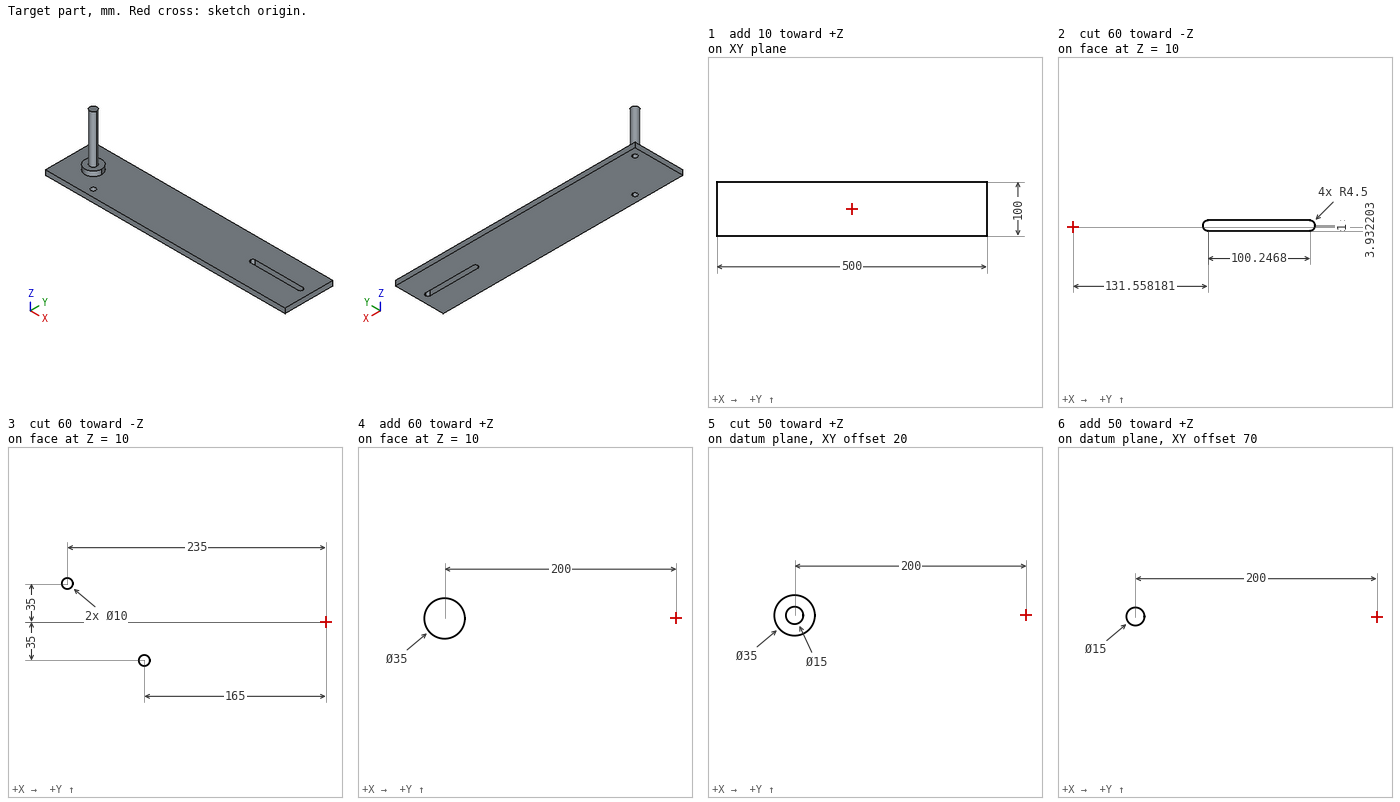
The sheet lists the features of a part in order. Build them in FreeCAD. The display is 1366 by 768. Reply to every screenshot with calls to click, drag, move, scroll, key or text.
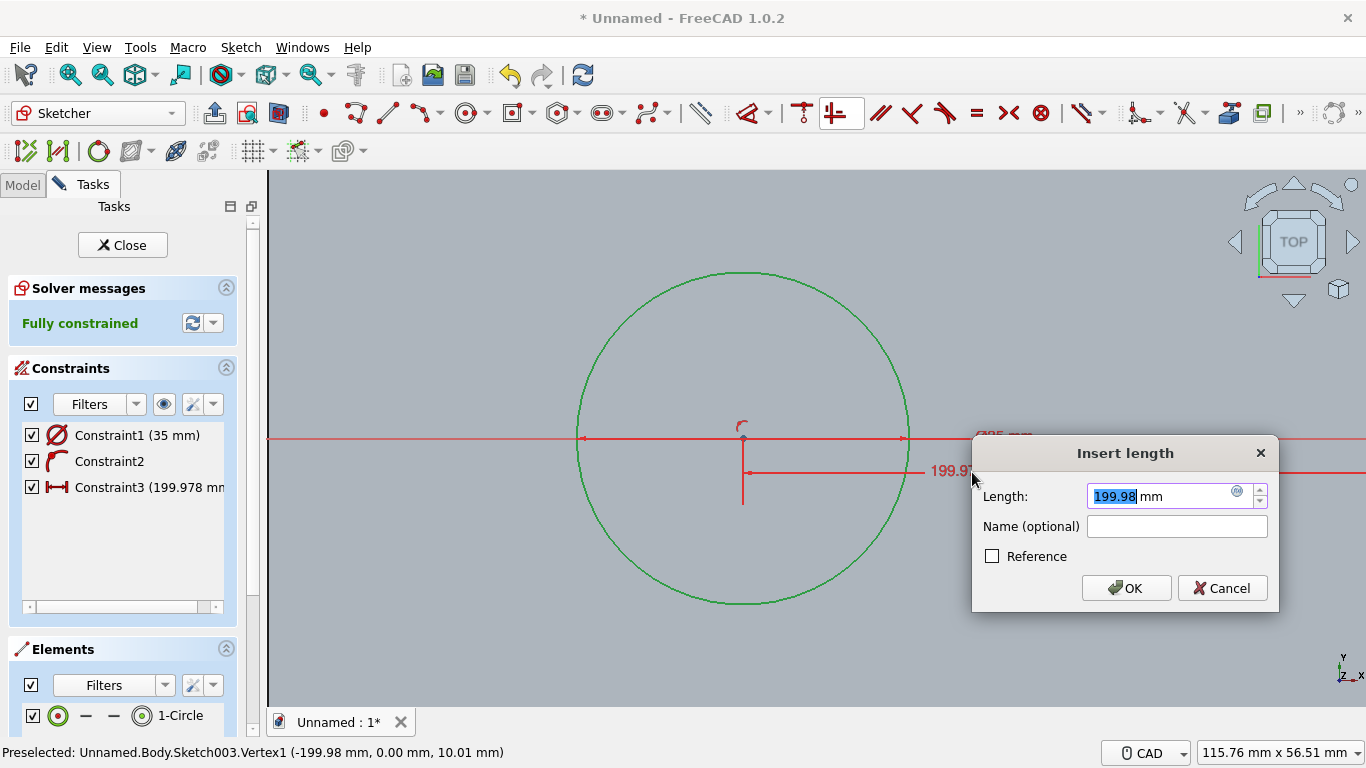
text(200)
key(Return)
key(Escape)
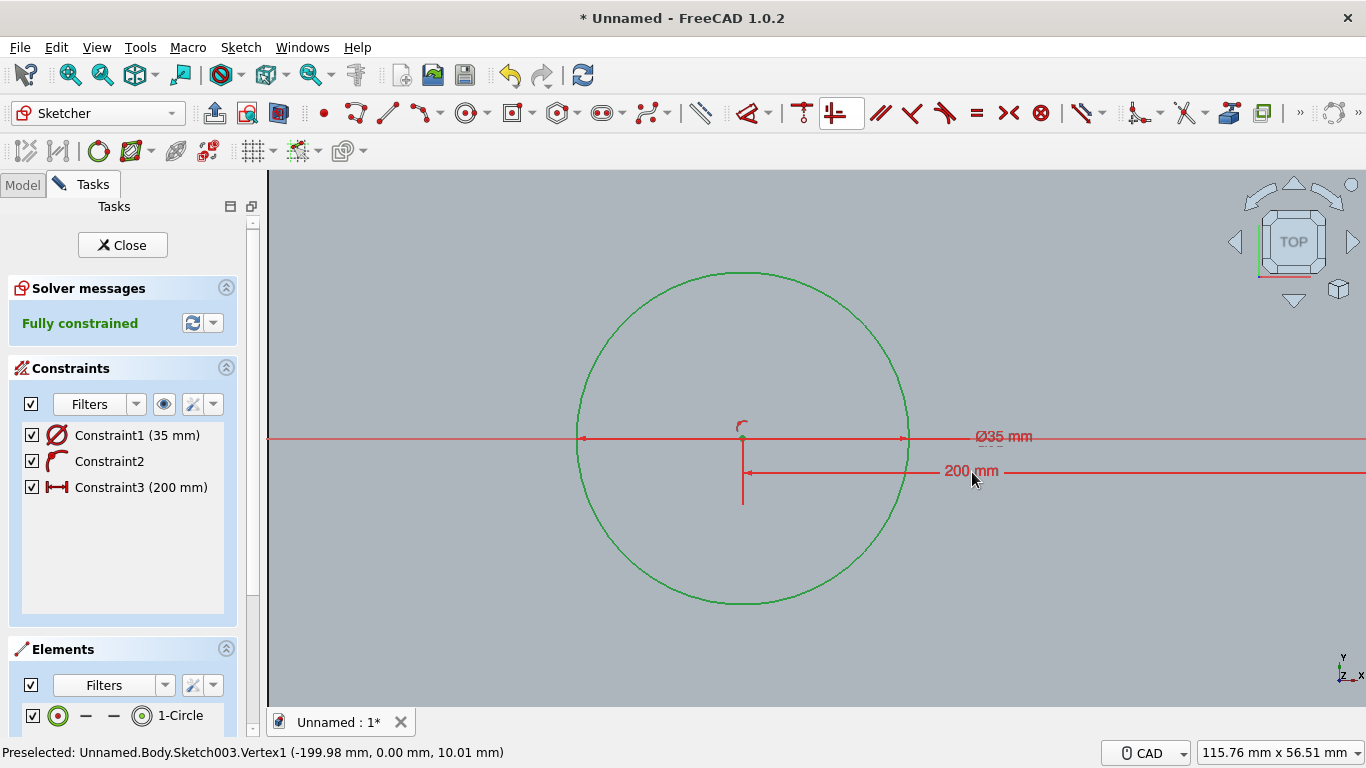
click(123, 245)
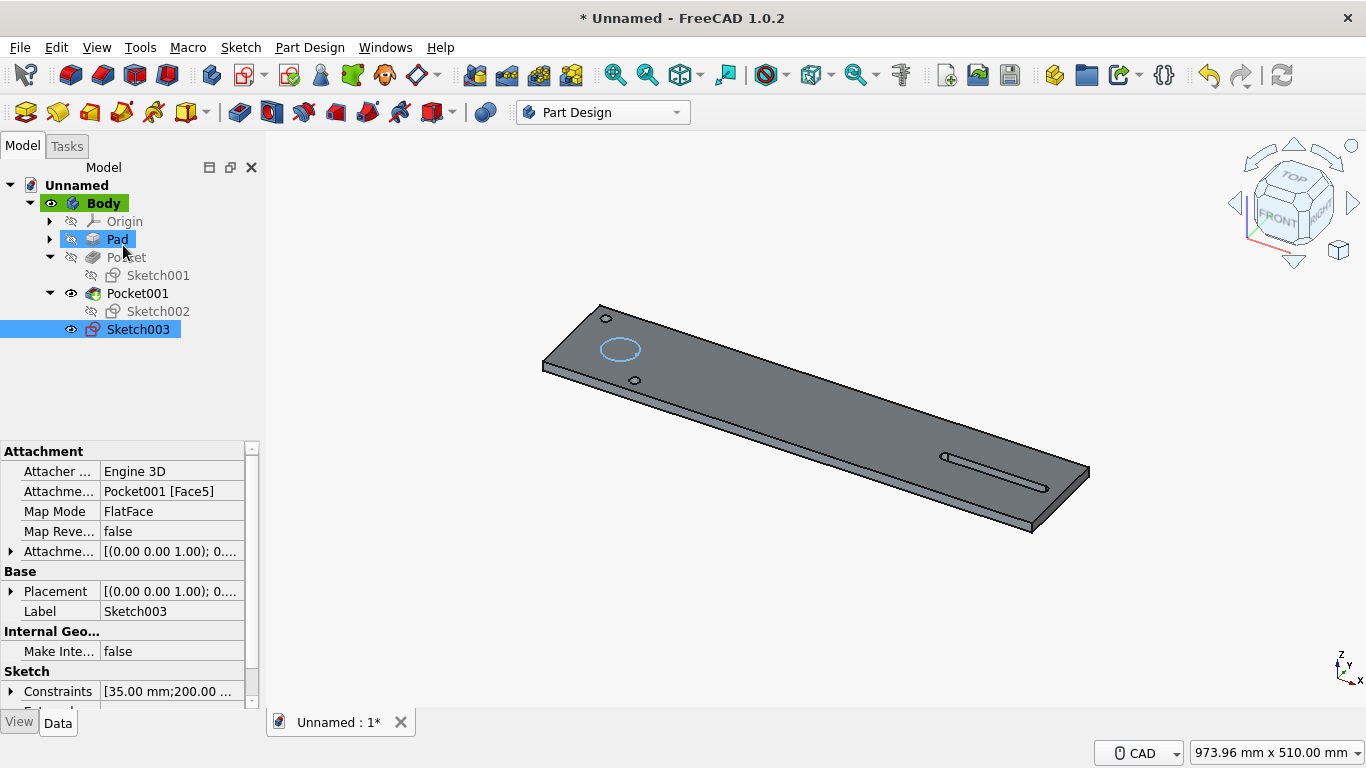
click(26, 112)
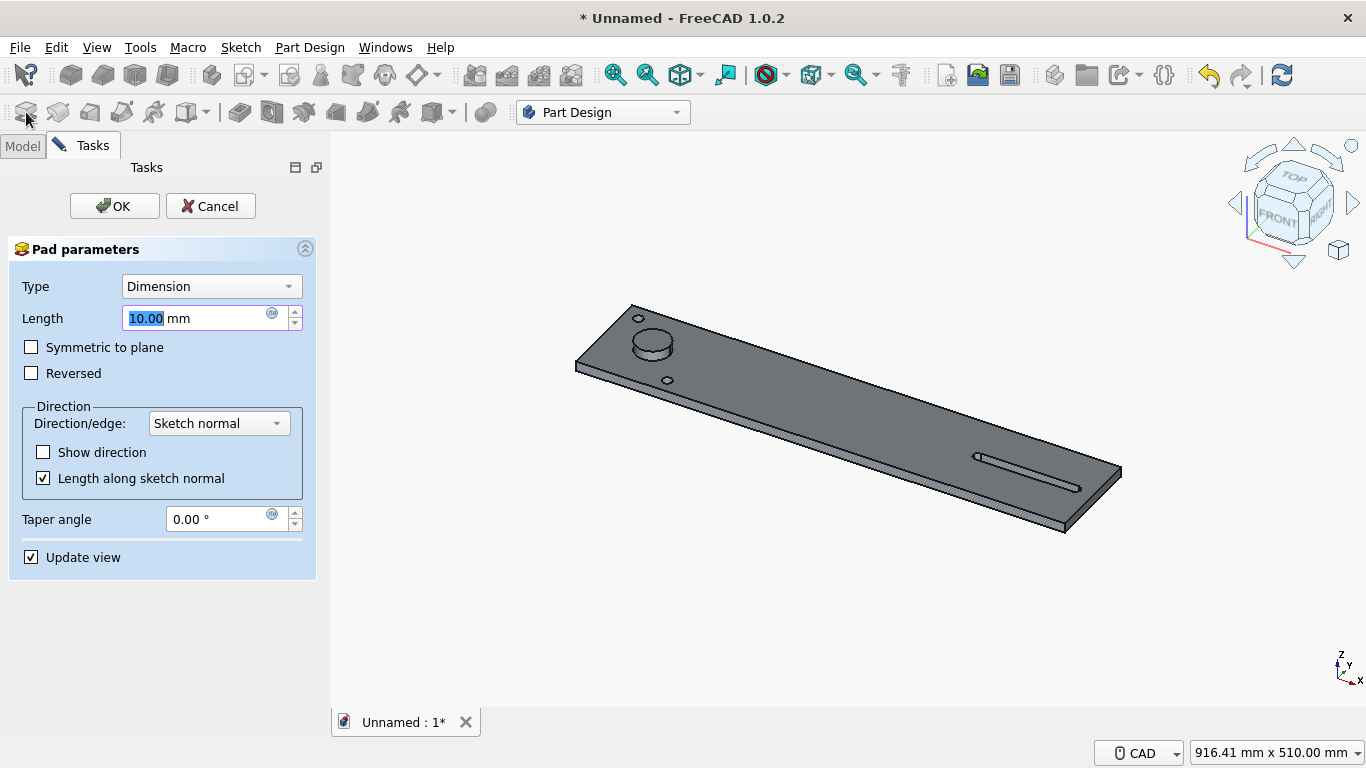
text(60)
key(Tab)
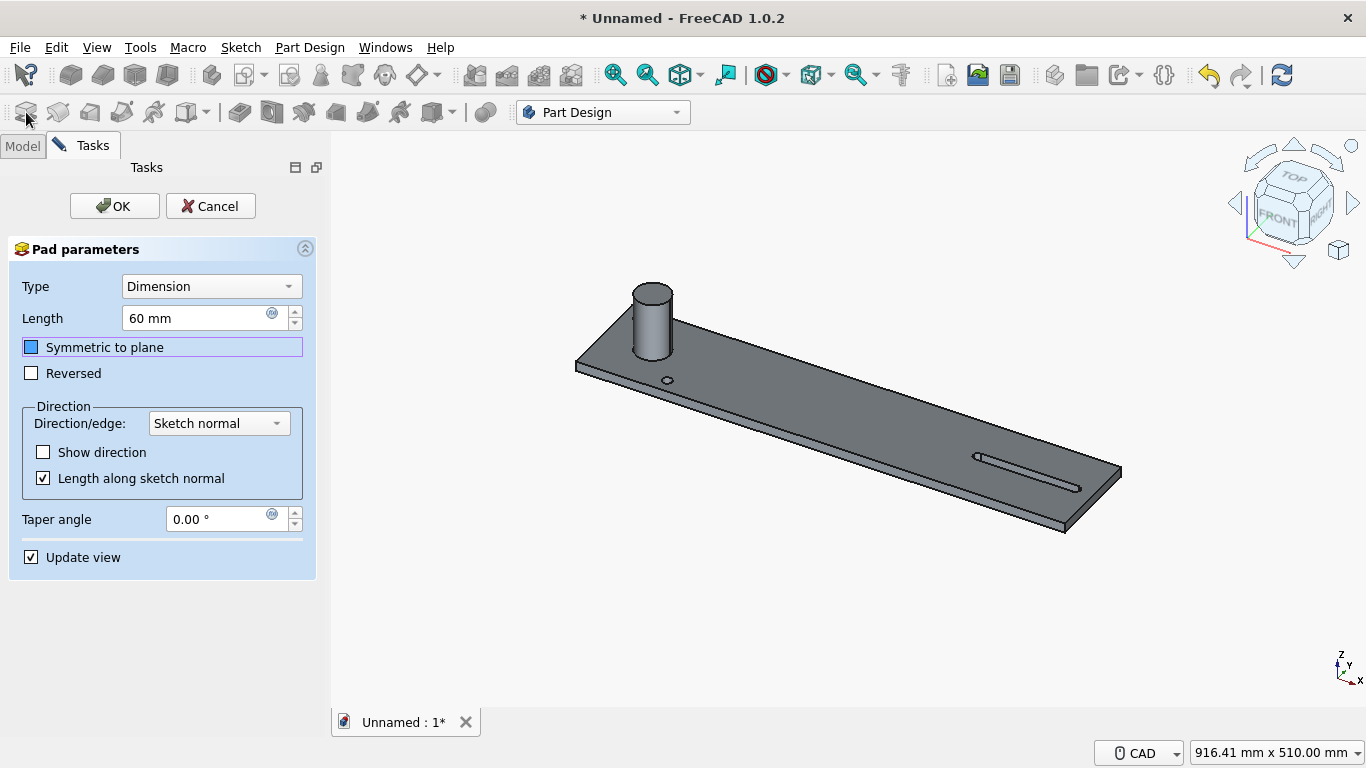
click(115, 206)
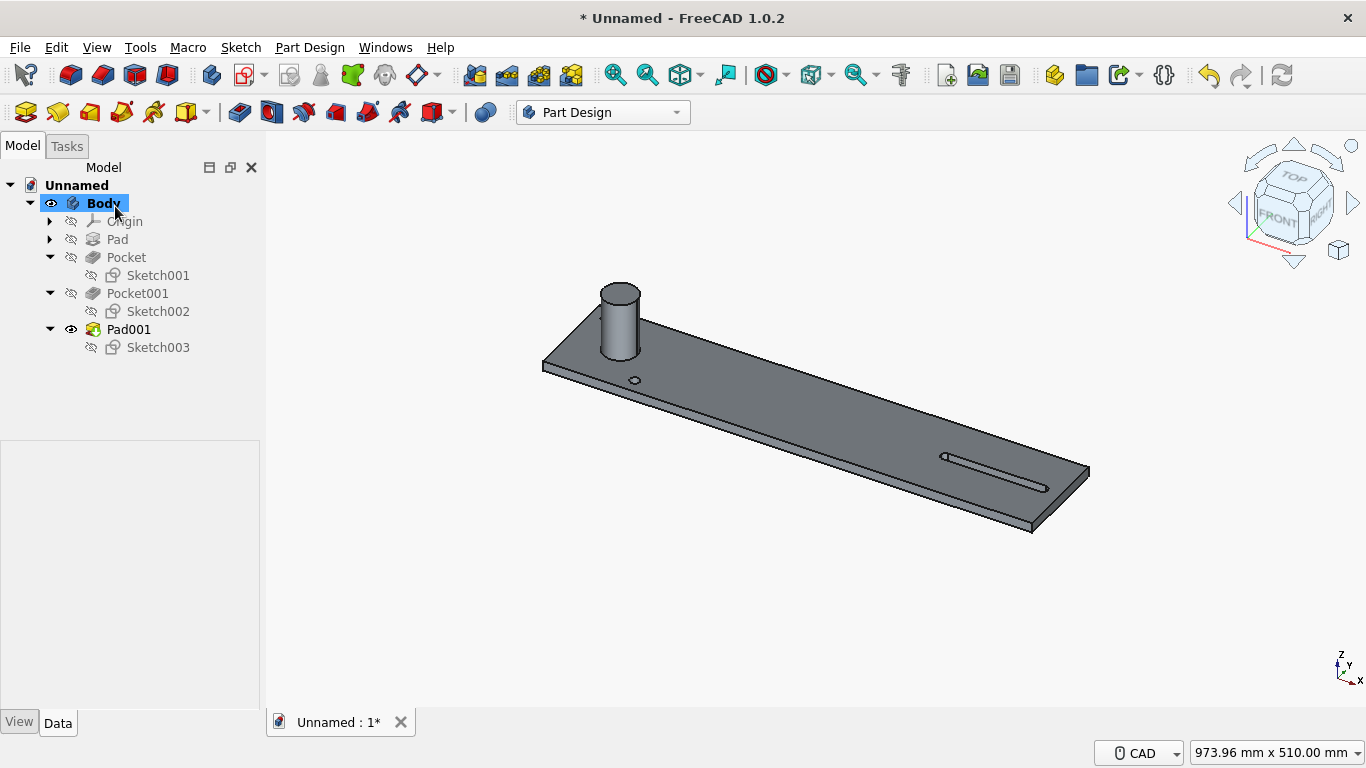
click(50, 221)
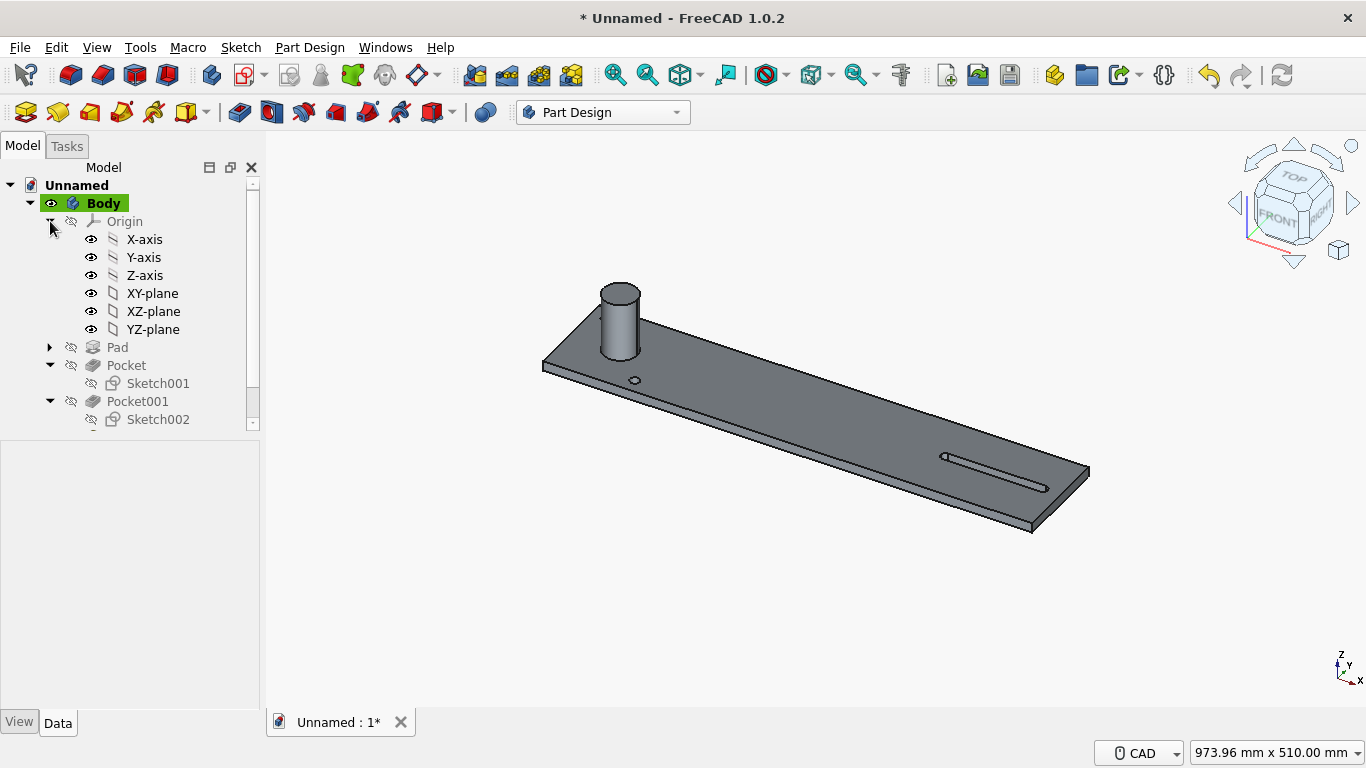
click(136, 293)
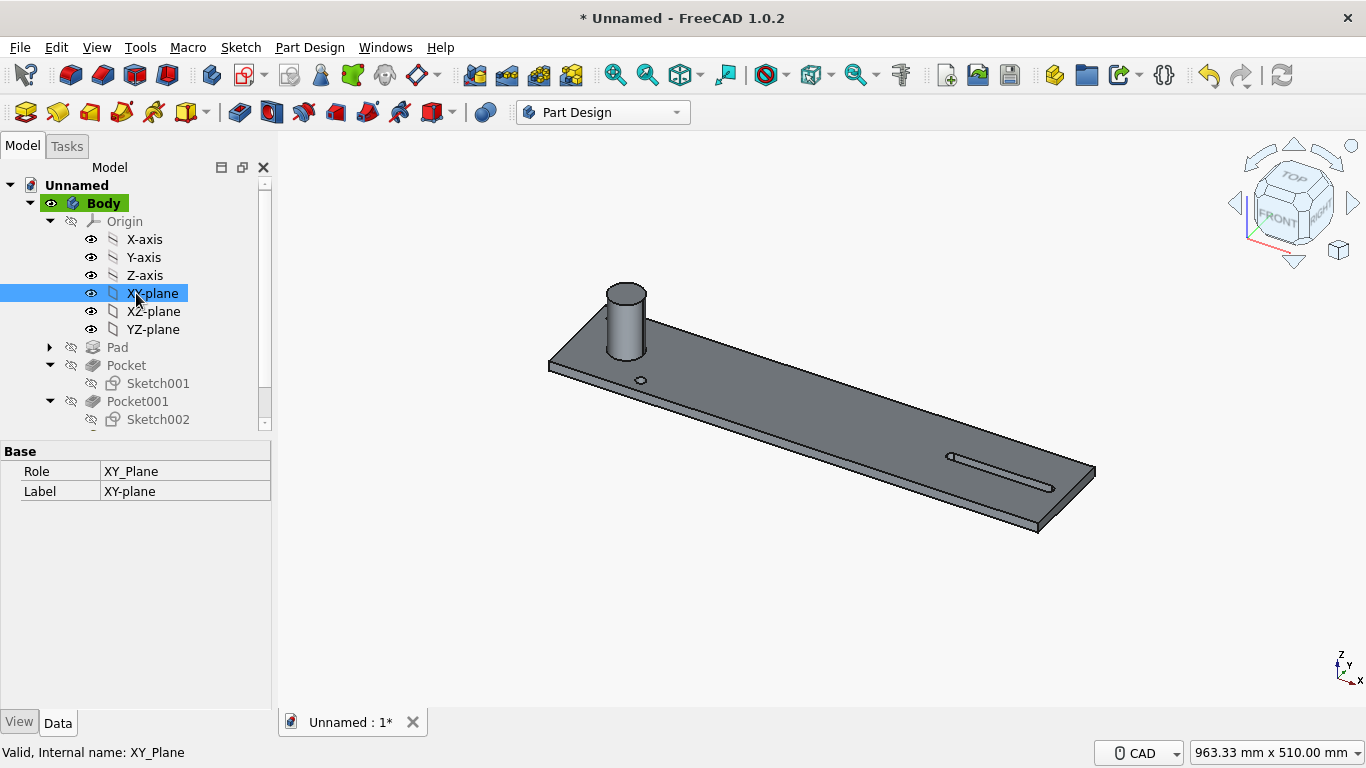
click(418, 76)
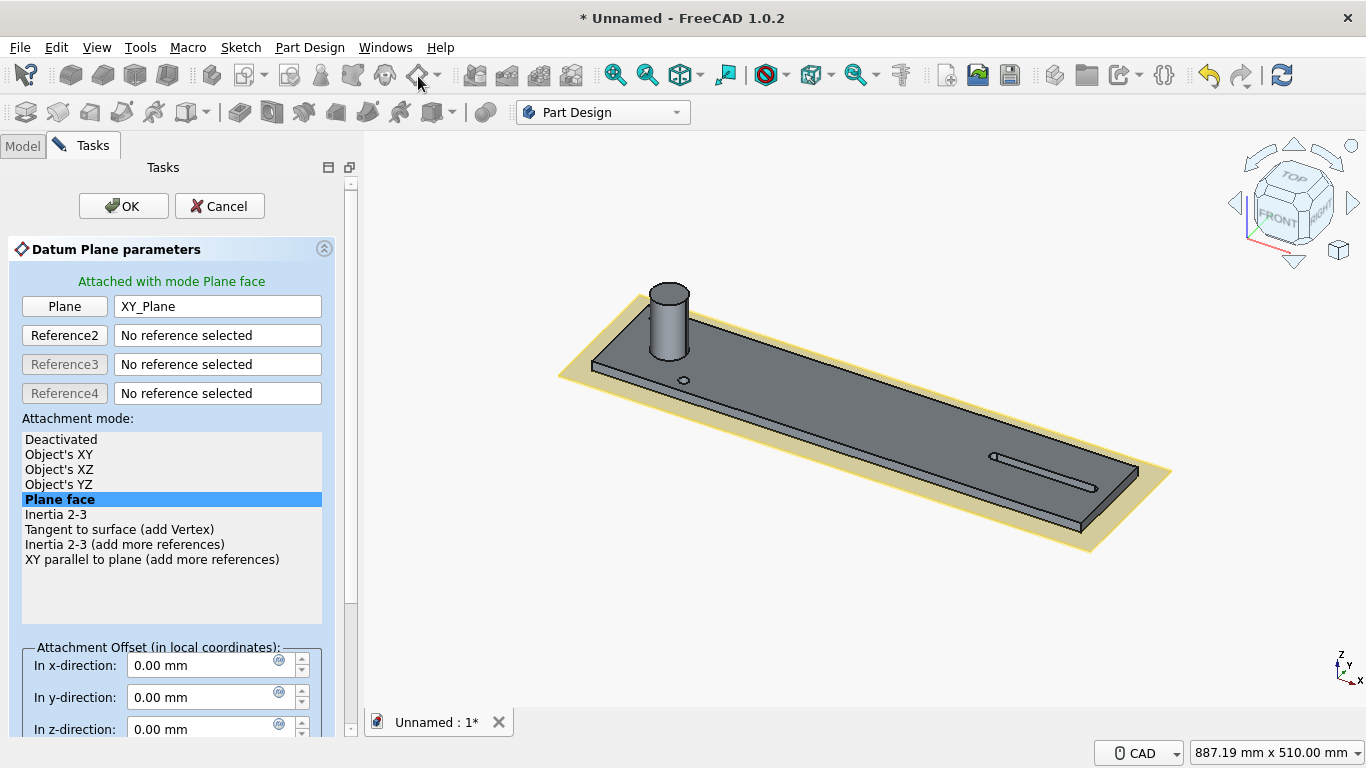
scroll(351, 456, down, 2)